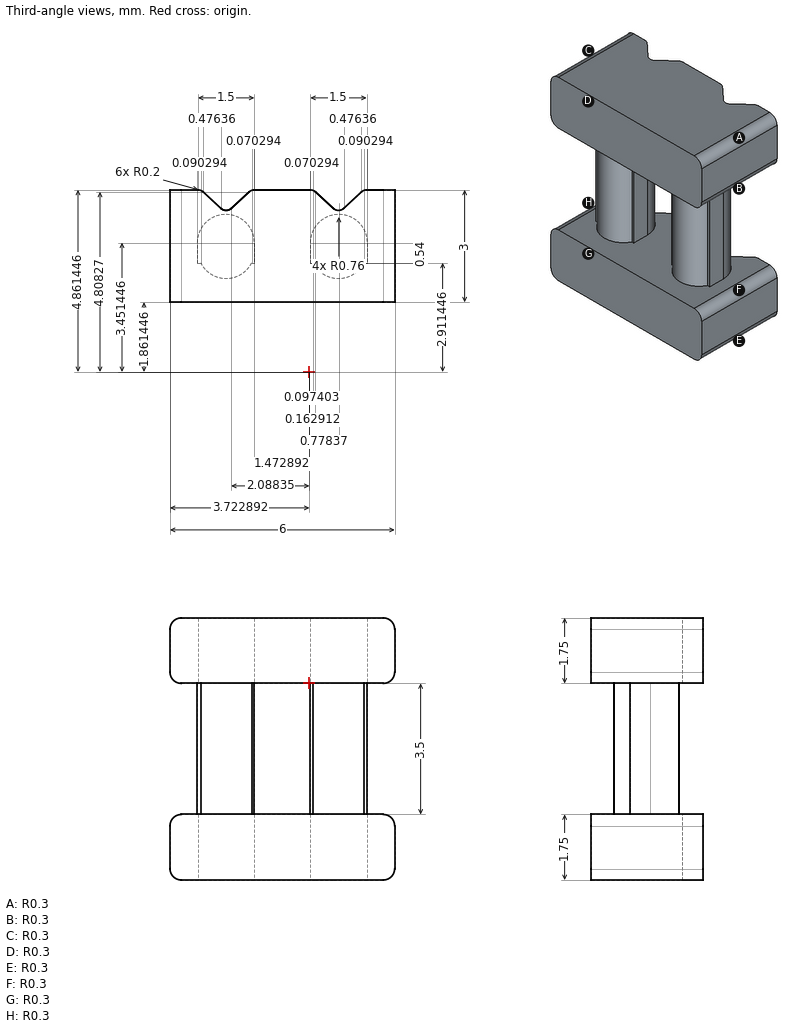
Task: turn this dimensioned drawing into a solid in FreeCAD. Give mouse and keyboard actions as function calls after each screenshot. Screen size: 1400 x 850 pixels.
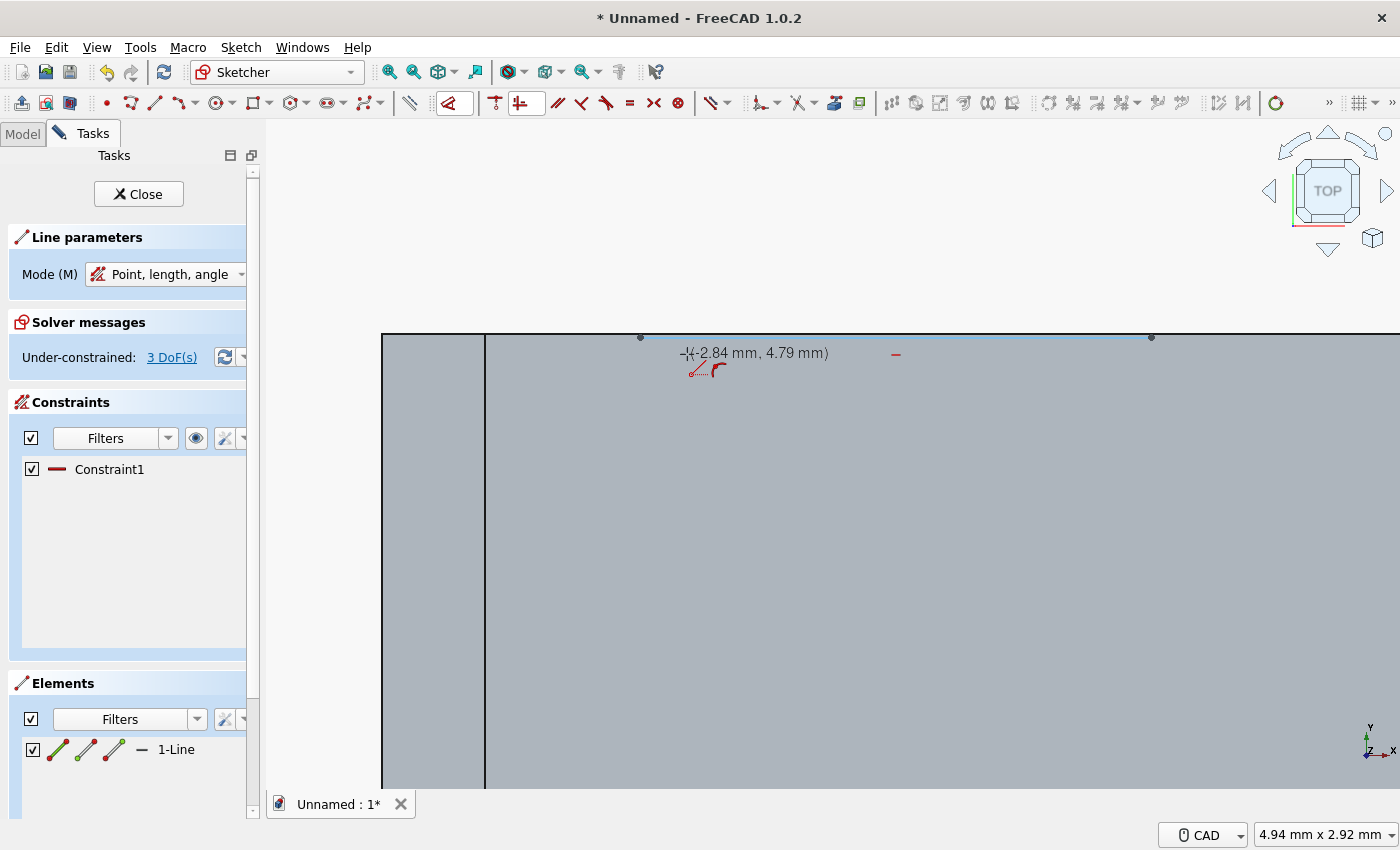
click(685, 353)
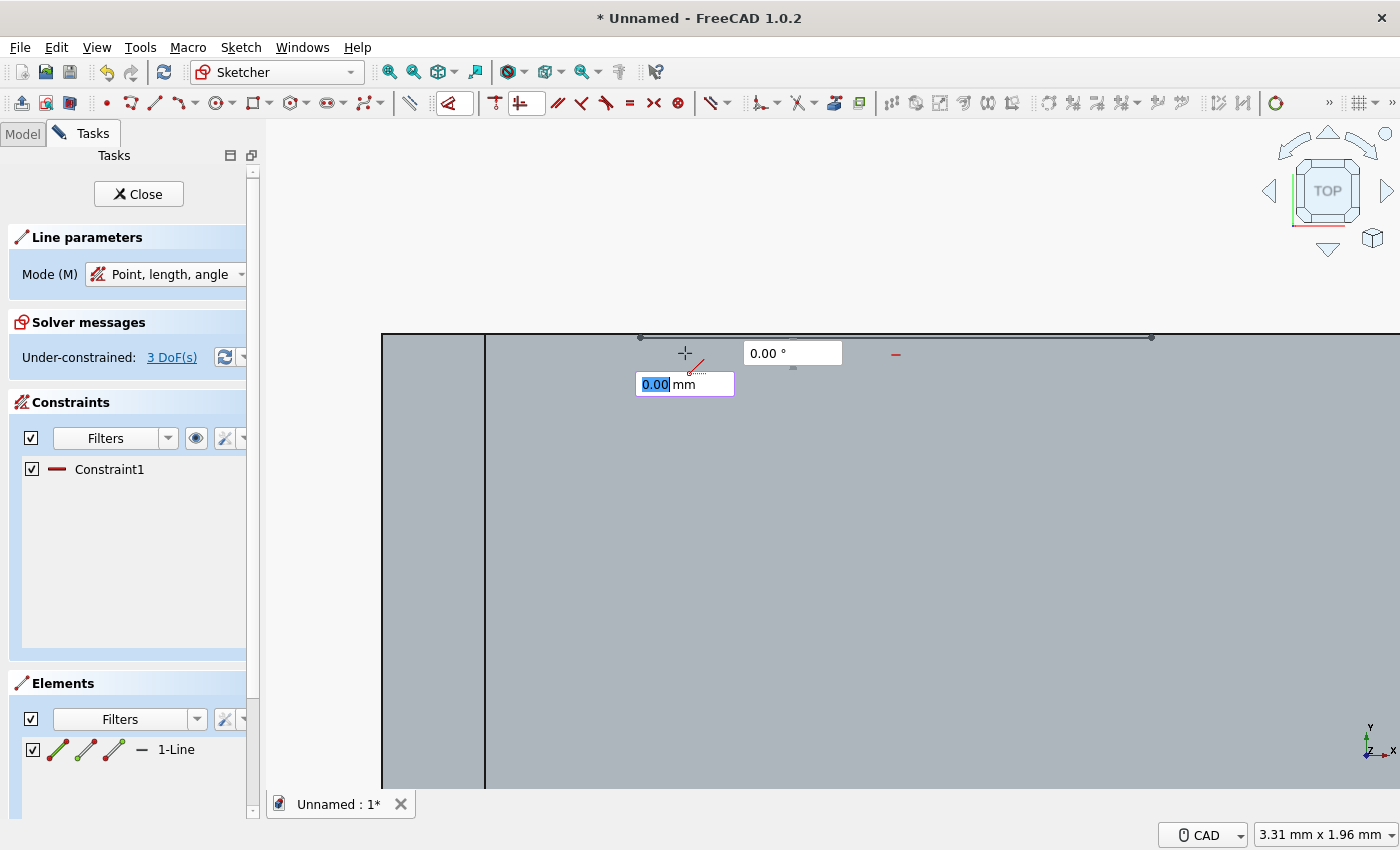
scroll(554, 221, down, 7)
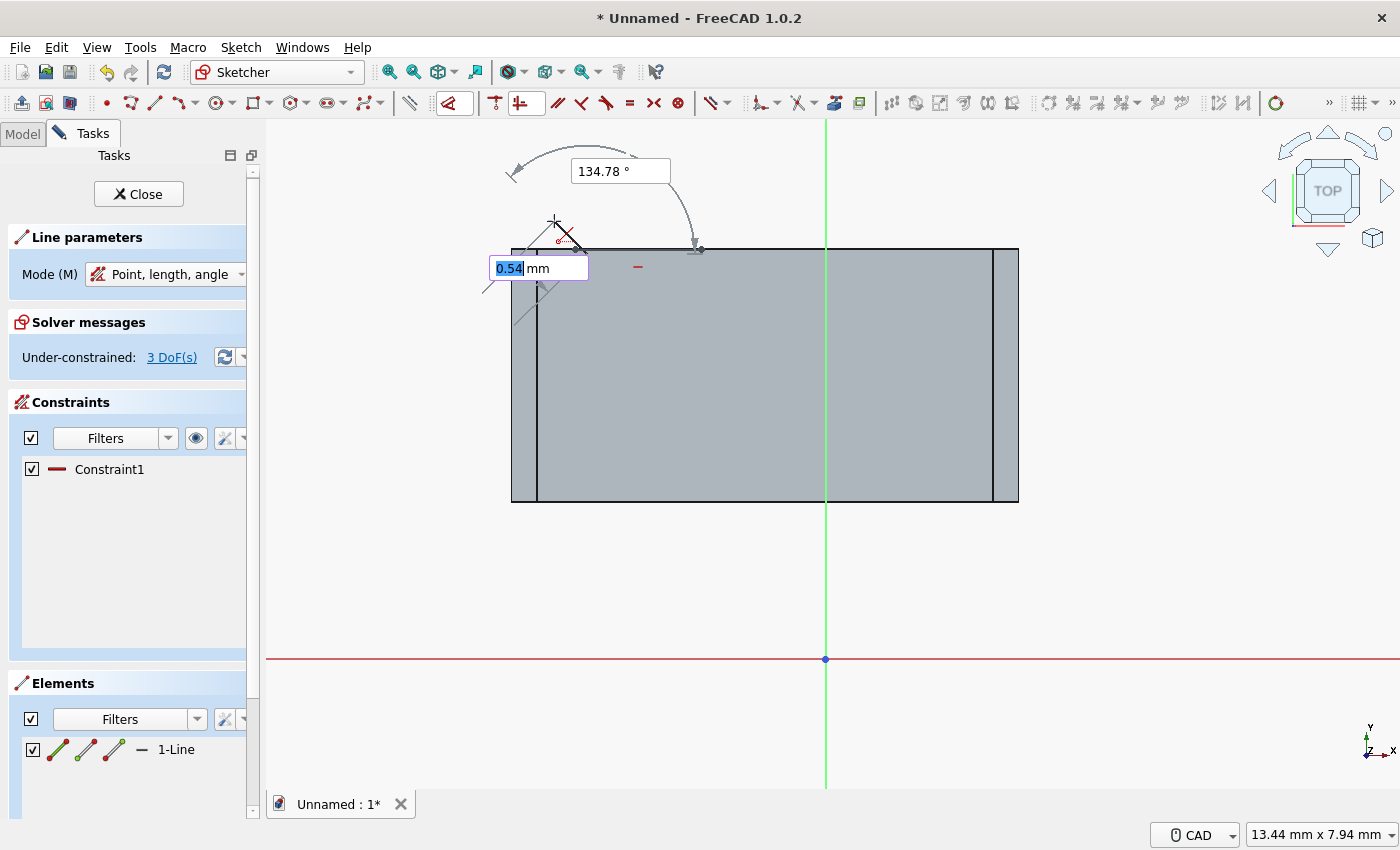
click(627, 291)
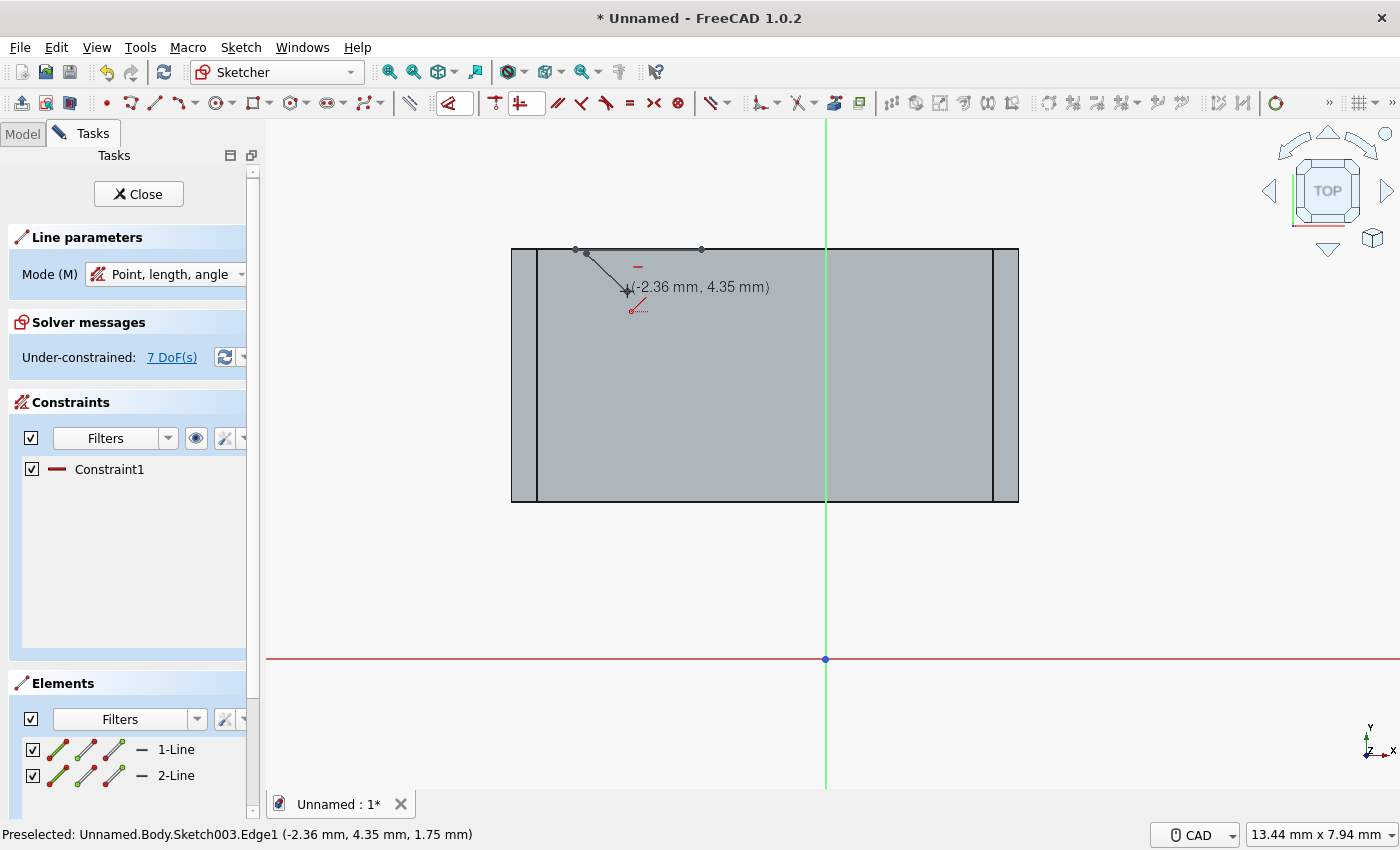
click(650, 291)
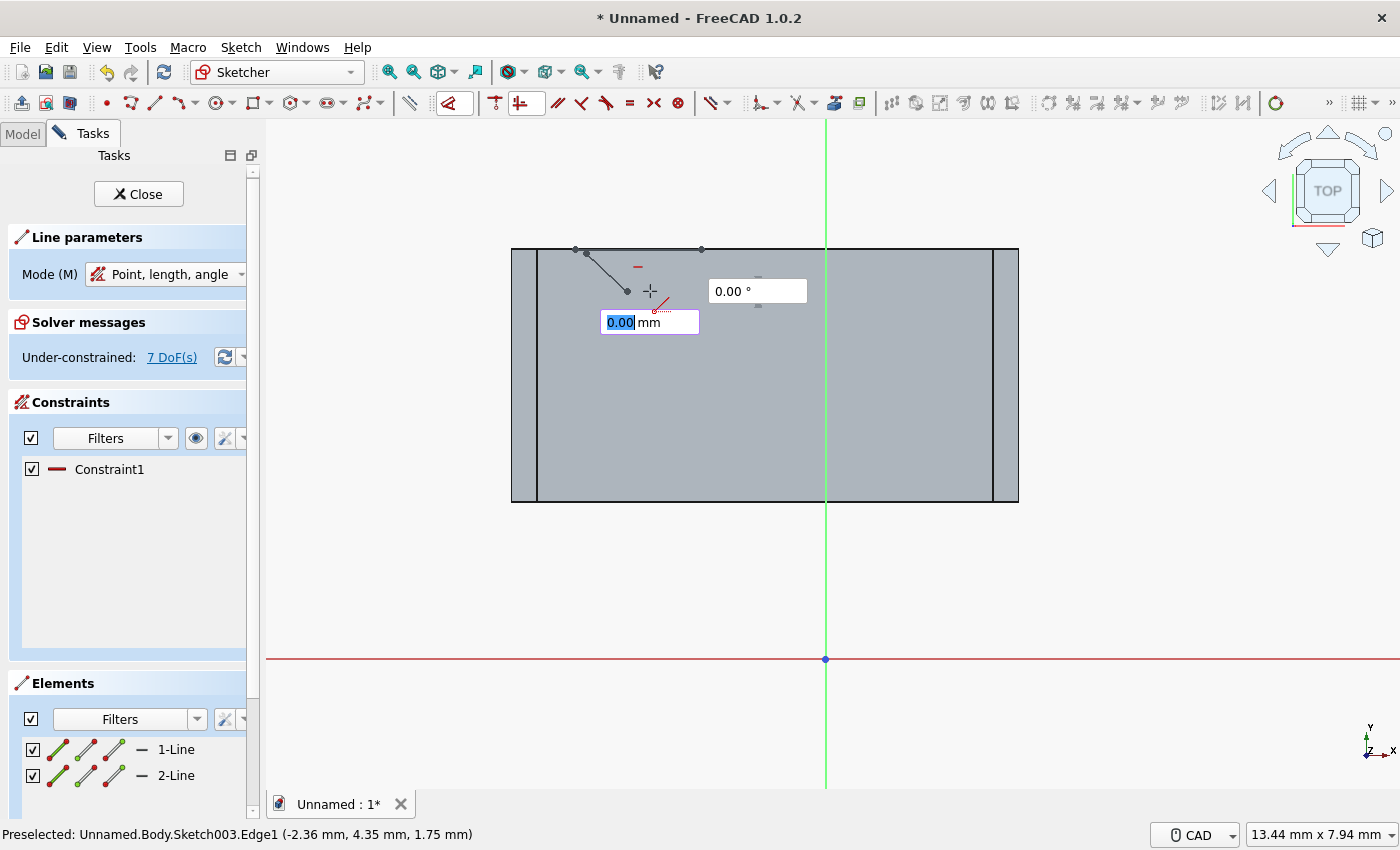
scroll(690, 254, up, 7)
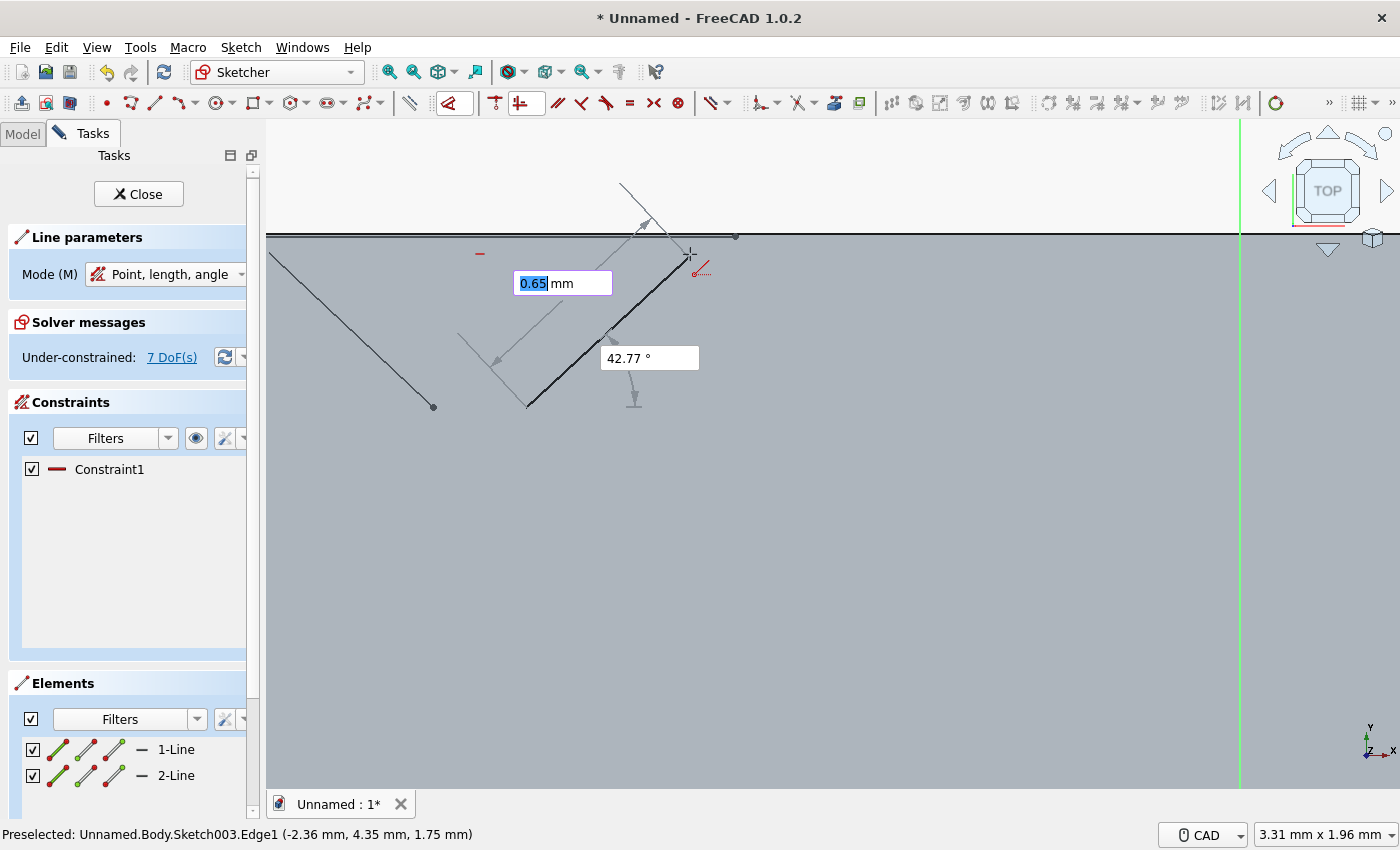
click(690, 252)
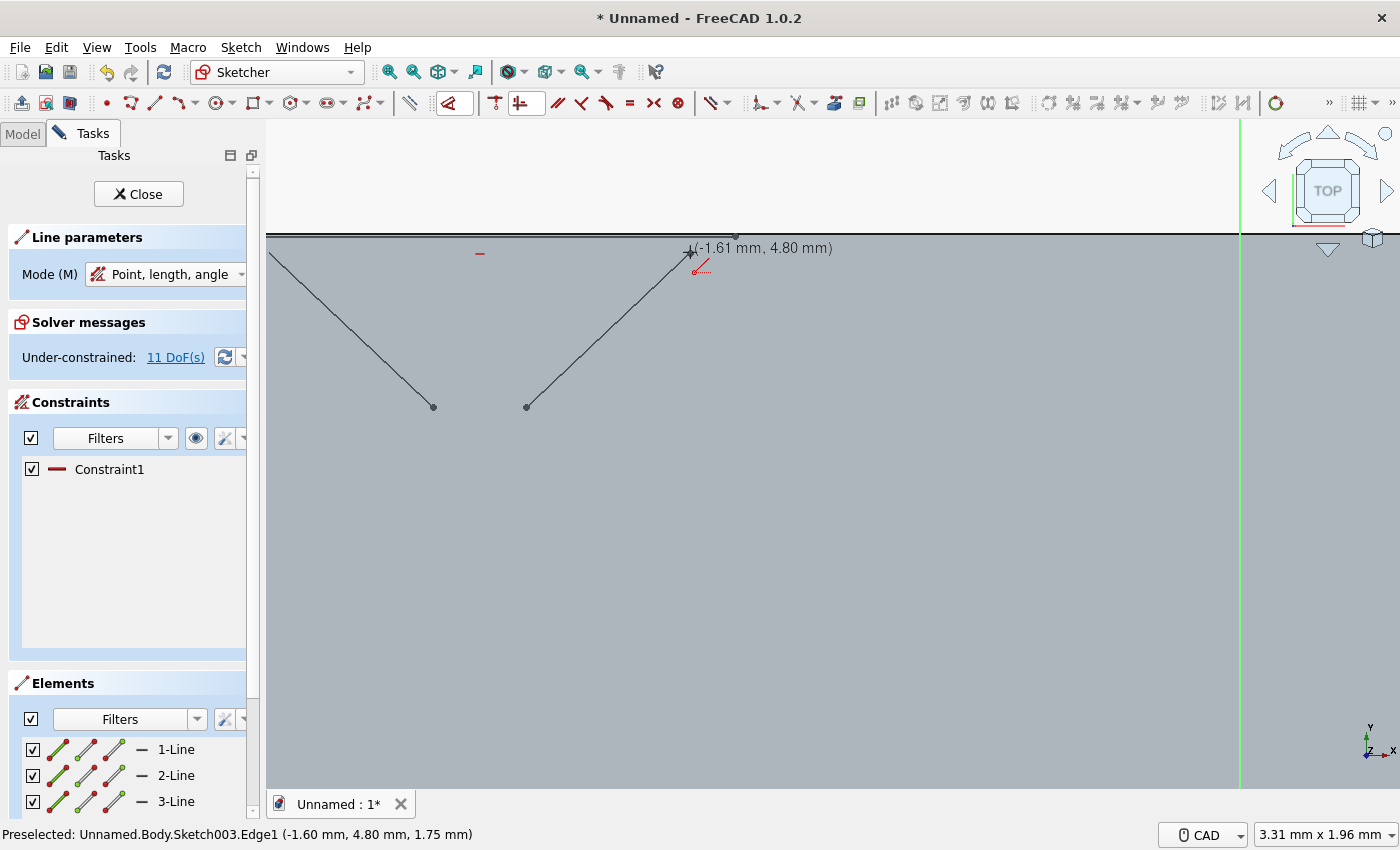
click(180, 104)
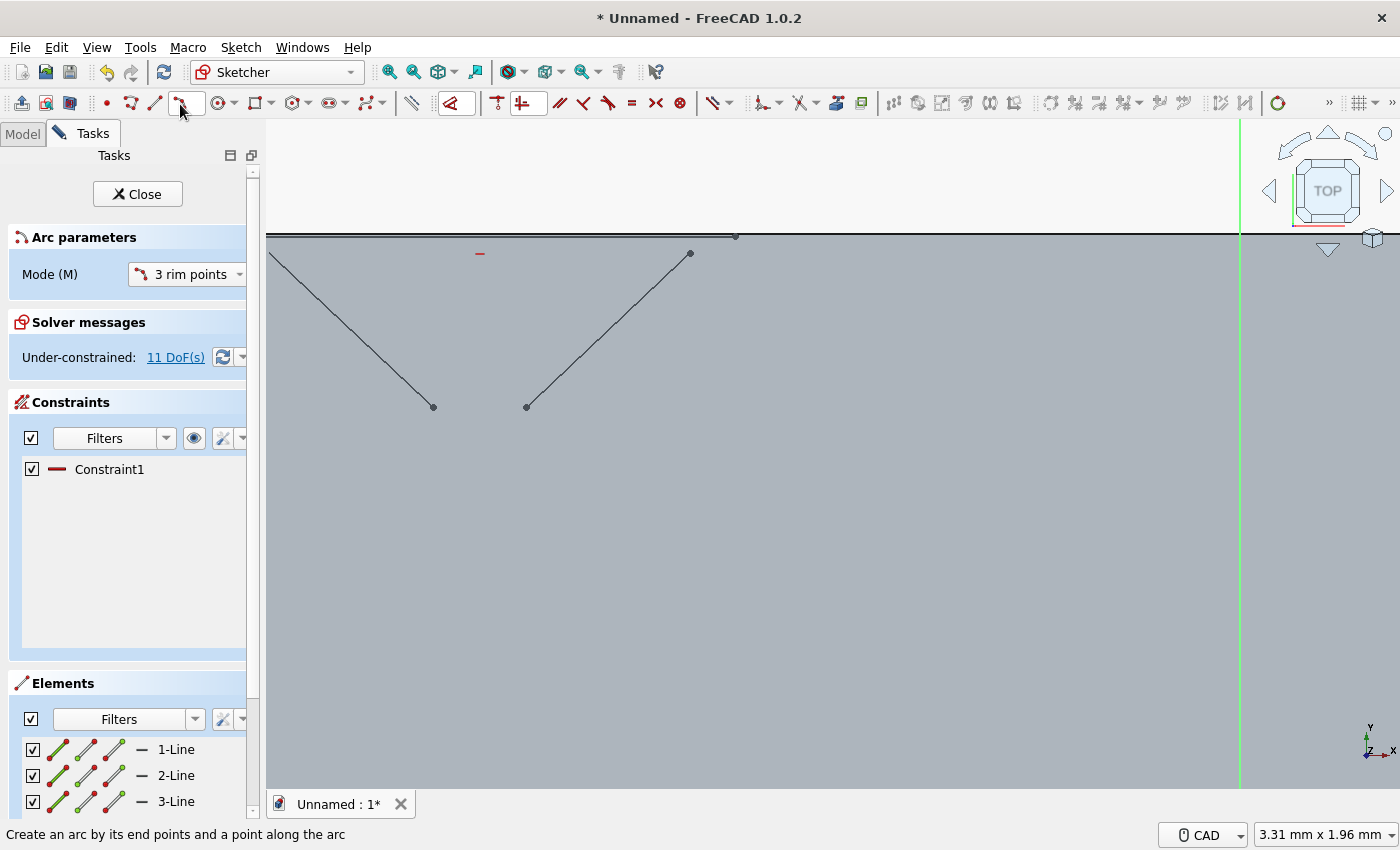
scroll(690, 254, down, 7)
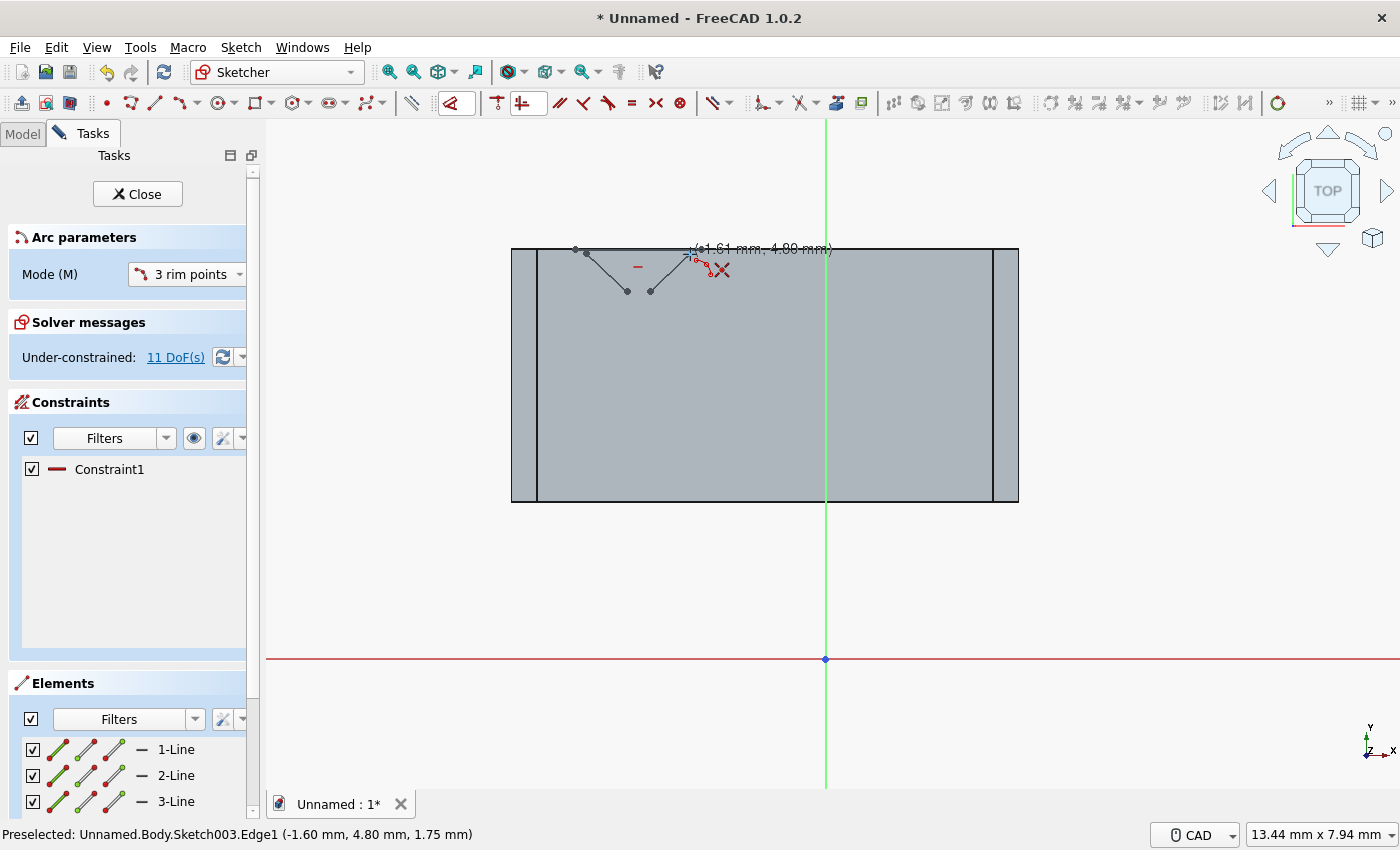
scroll(575, 249, up, 2)